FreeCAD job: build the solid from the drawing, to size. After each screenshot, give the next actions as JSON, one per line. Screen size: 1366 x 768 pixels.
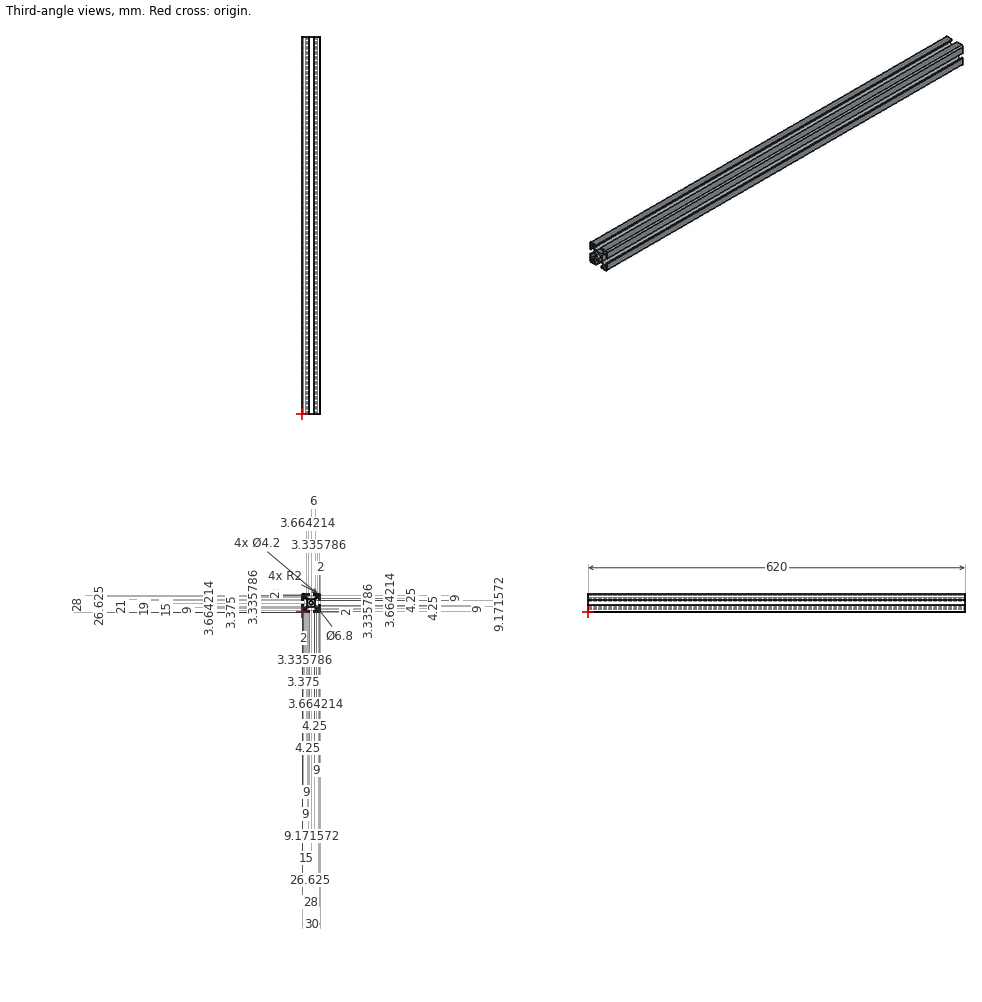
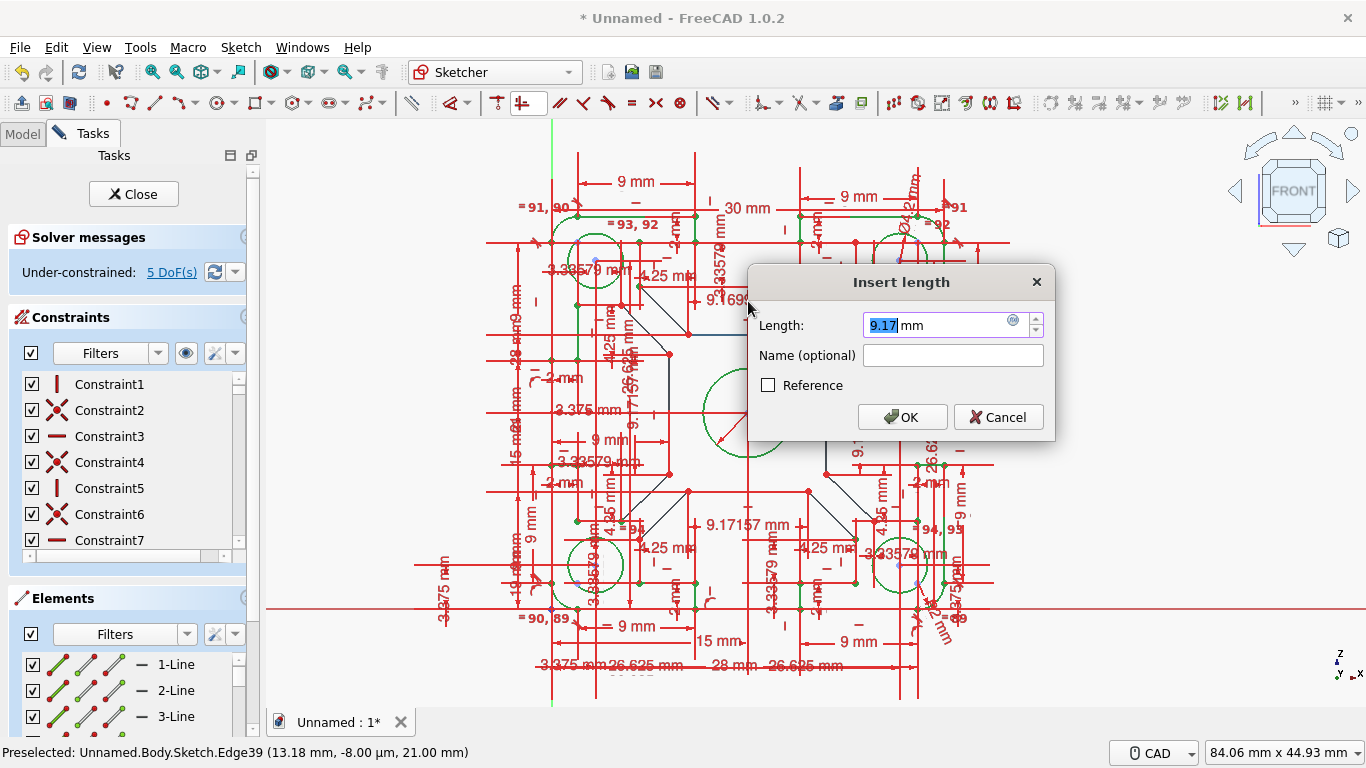
{"action": "type", "text": "9.171572"}
{"action": "key", "text": "Return"}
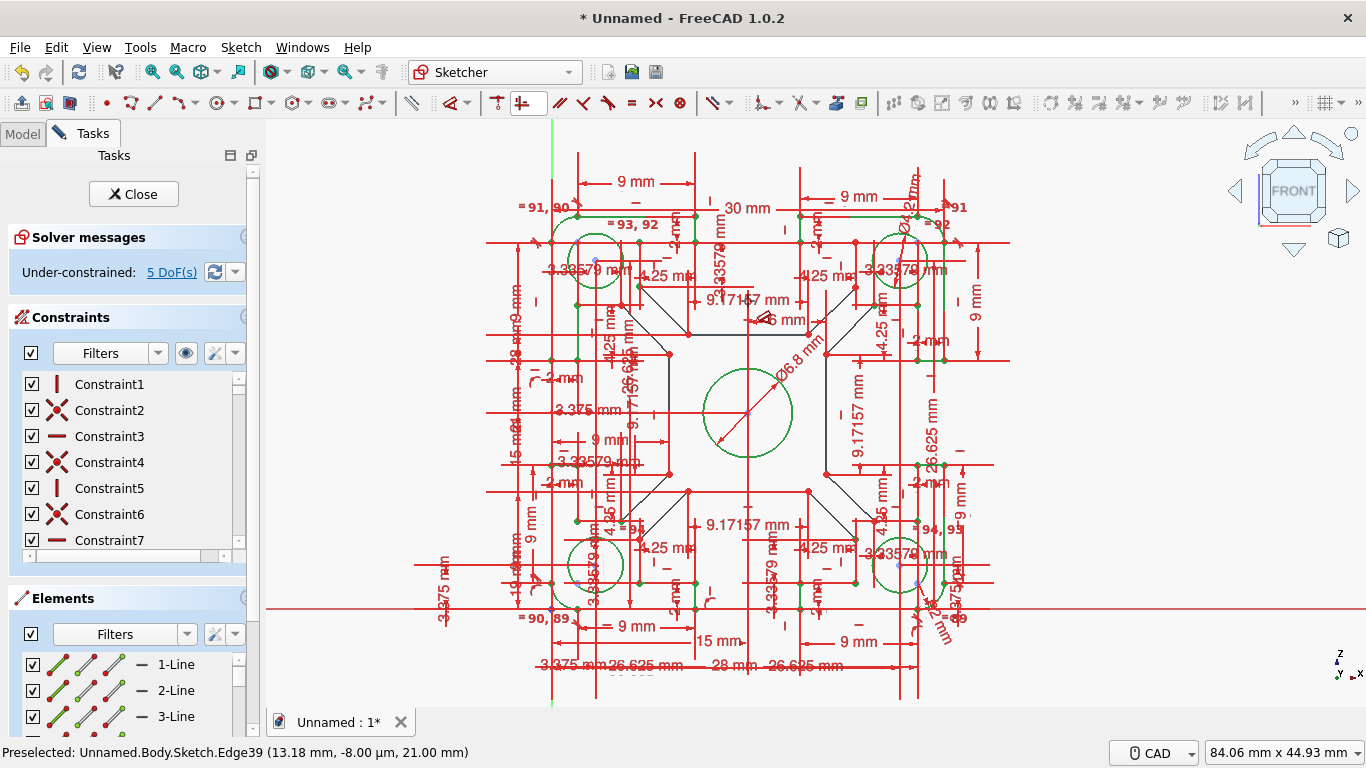
{"action": "left_click", "coordinate": [856, 274]}
{"action": "left_click", "coordinate": [962, 250]}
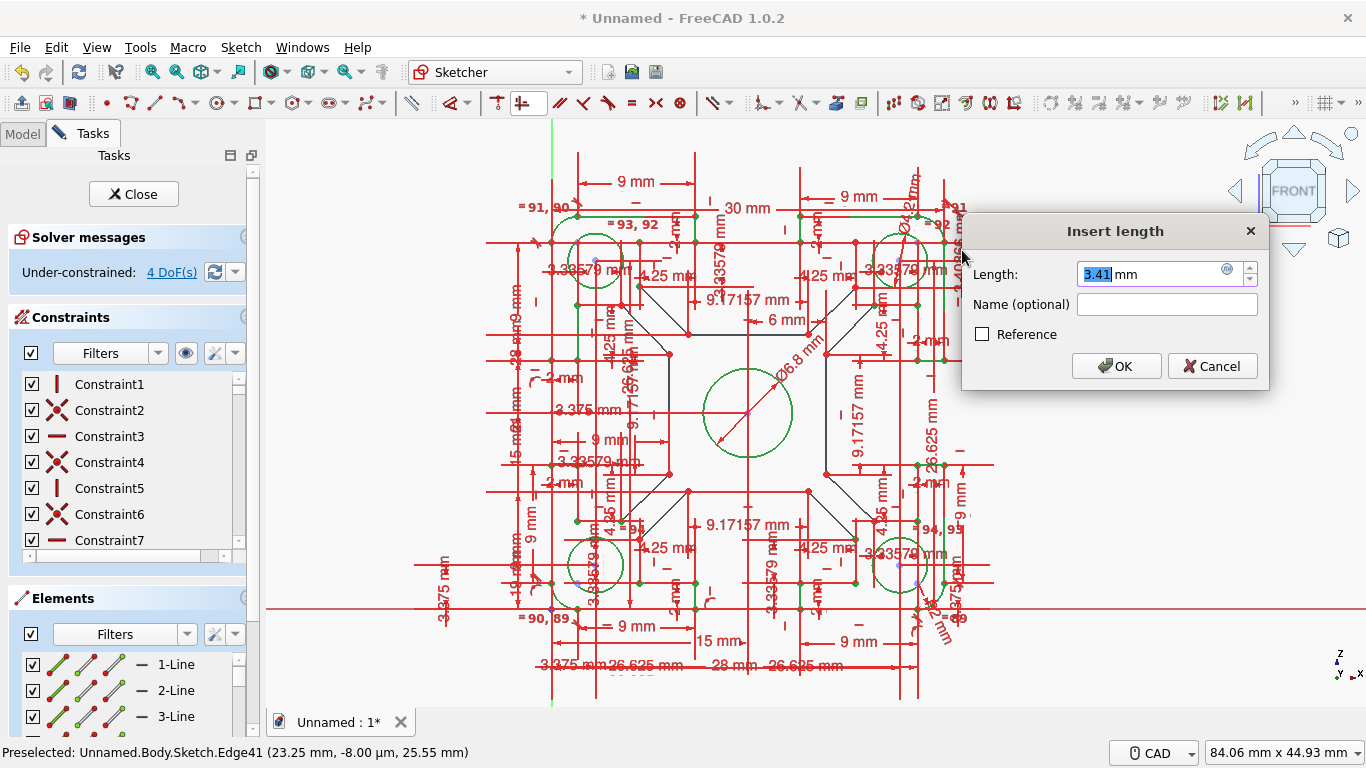
{"action": "type", "text": "3.335786"}
{"action": "key", "text": "Return"}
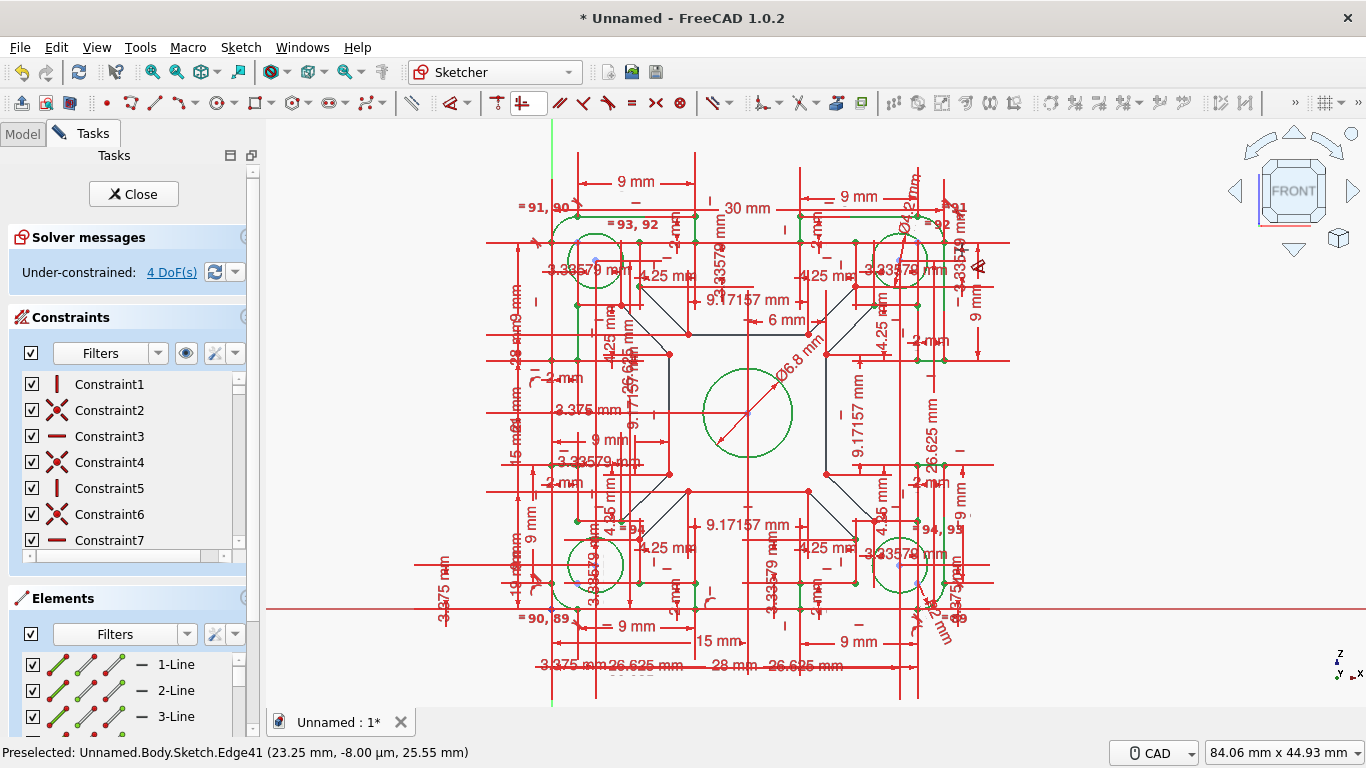
{"action": "left_click", "coordinate": [860, 320]}
{"action": "left_click", "coordinate": [1004, 330]}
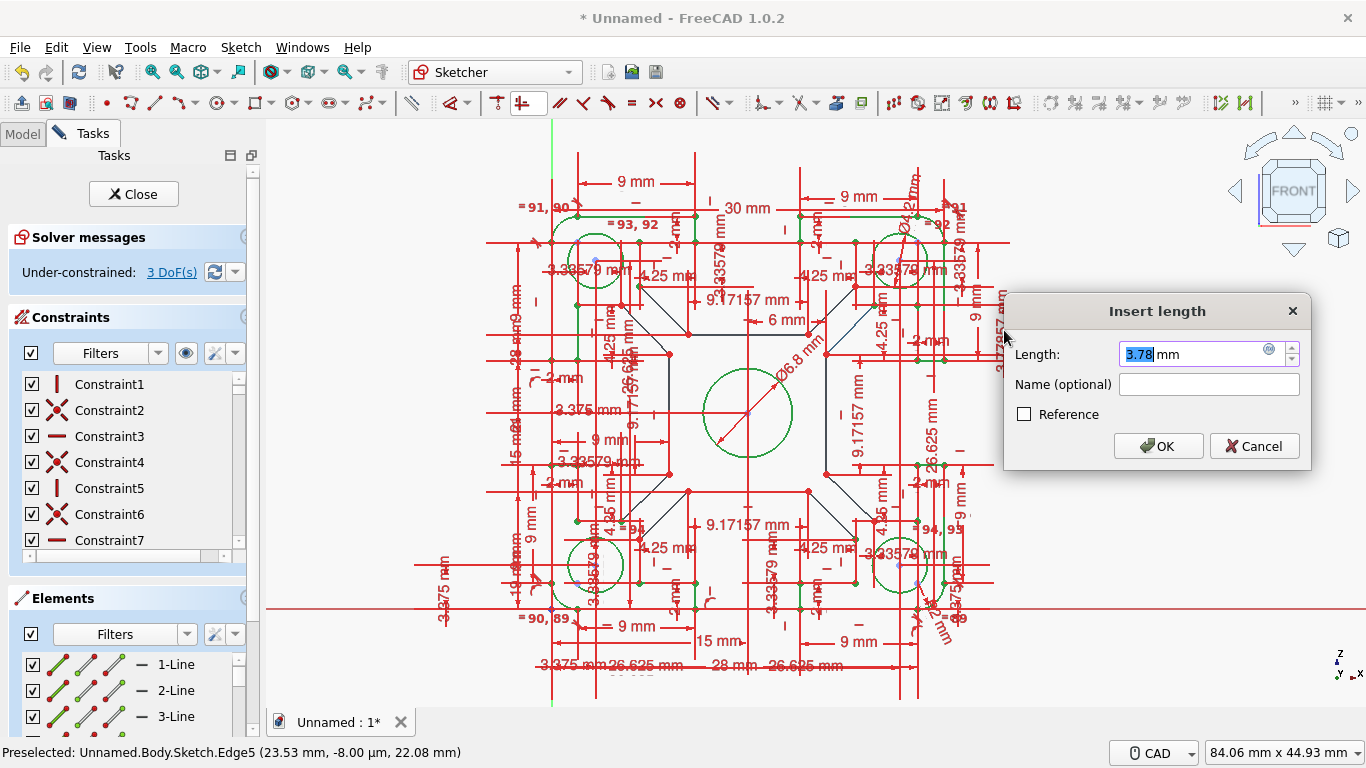
{"action": "type", "text": "3.664214"}
{"action": "key", "text": "Return"}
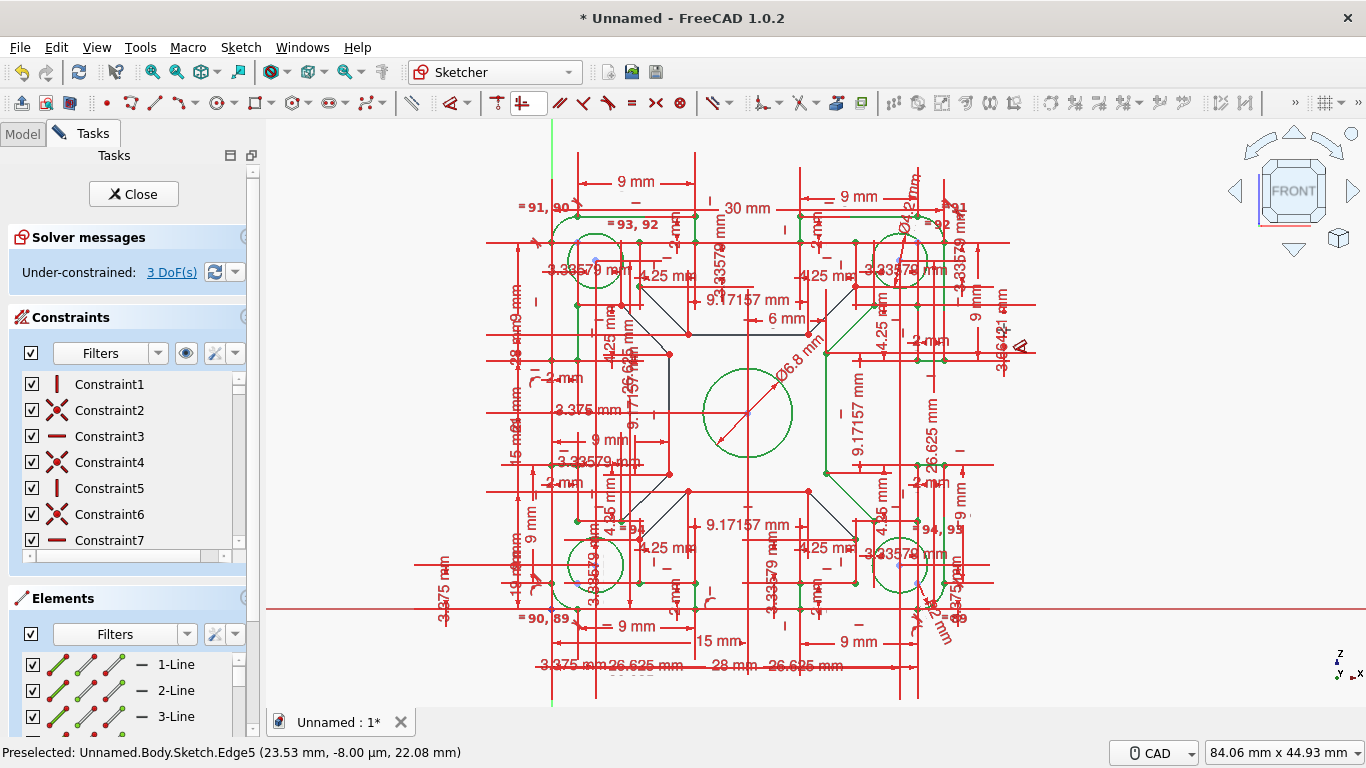
{"action": "left_click", "coordinate": [841, 525]}
{"action": "left_click", "coordinate": [843, 458]}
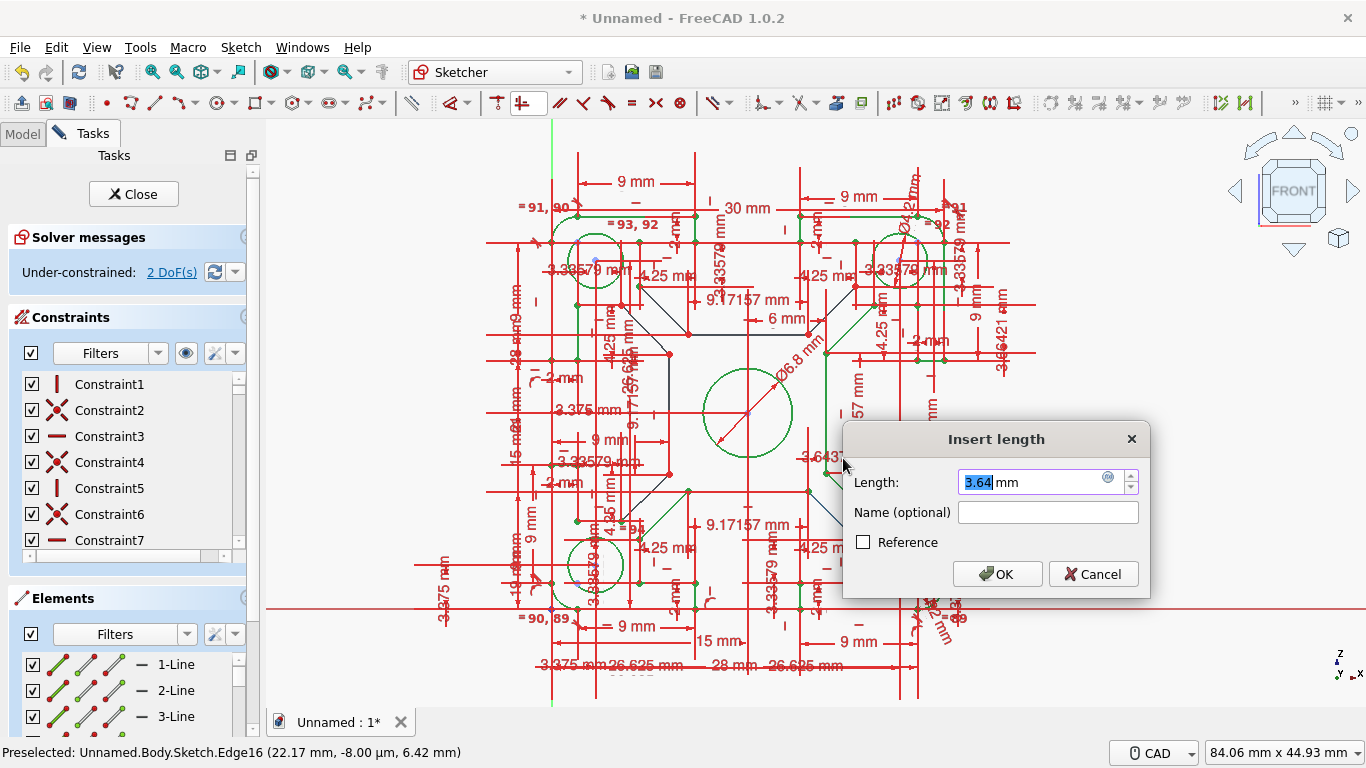
{"action": "type", "text": "3.664214"}
{"action": "key", "text": "Return"}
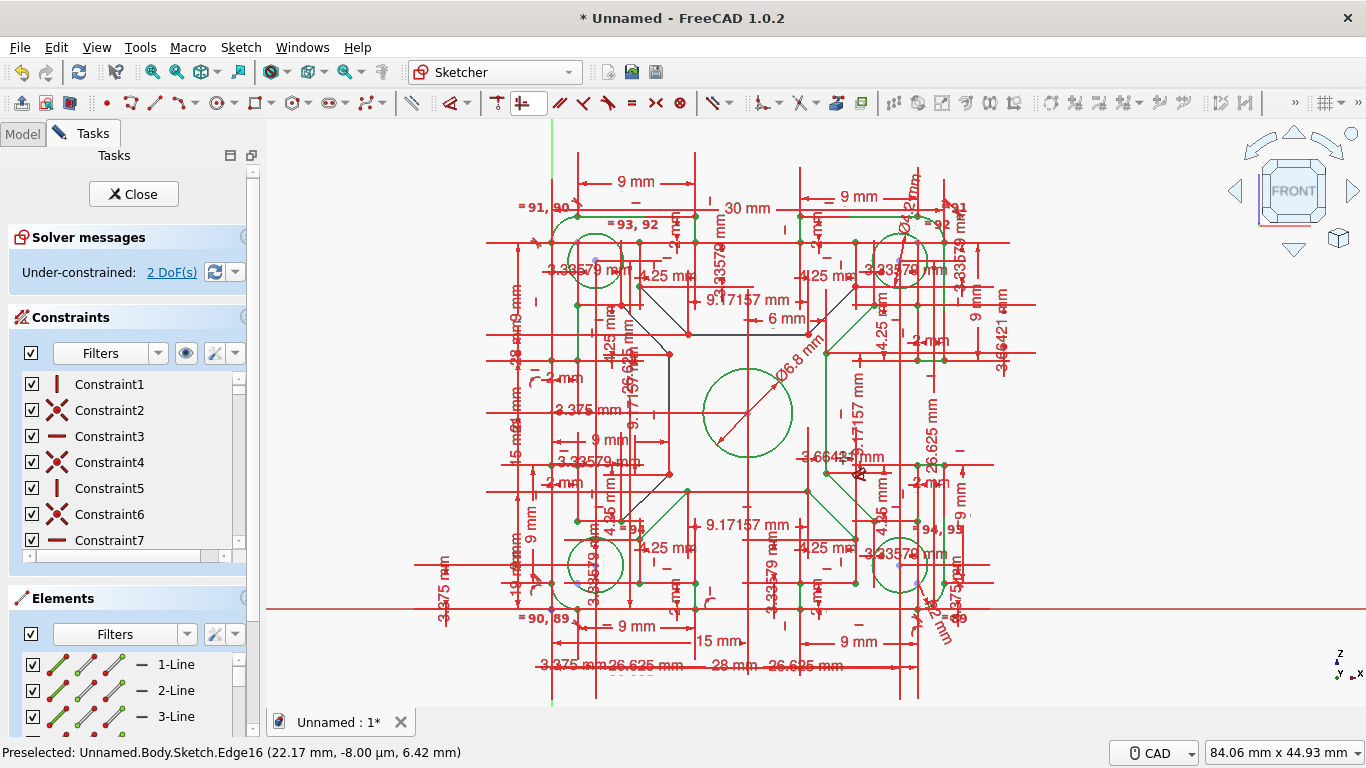
{"action": "left_click", "coordinate": [636, 507]}
{"action": "left_click", "coordinate": [491, 498]}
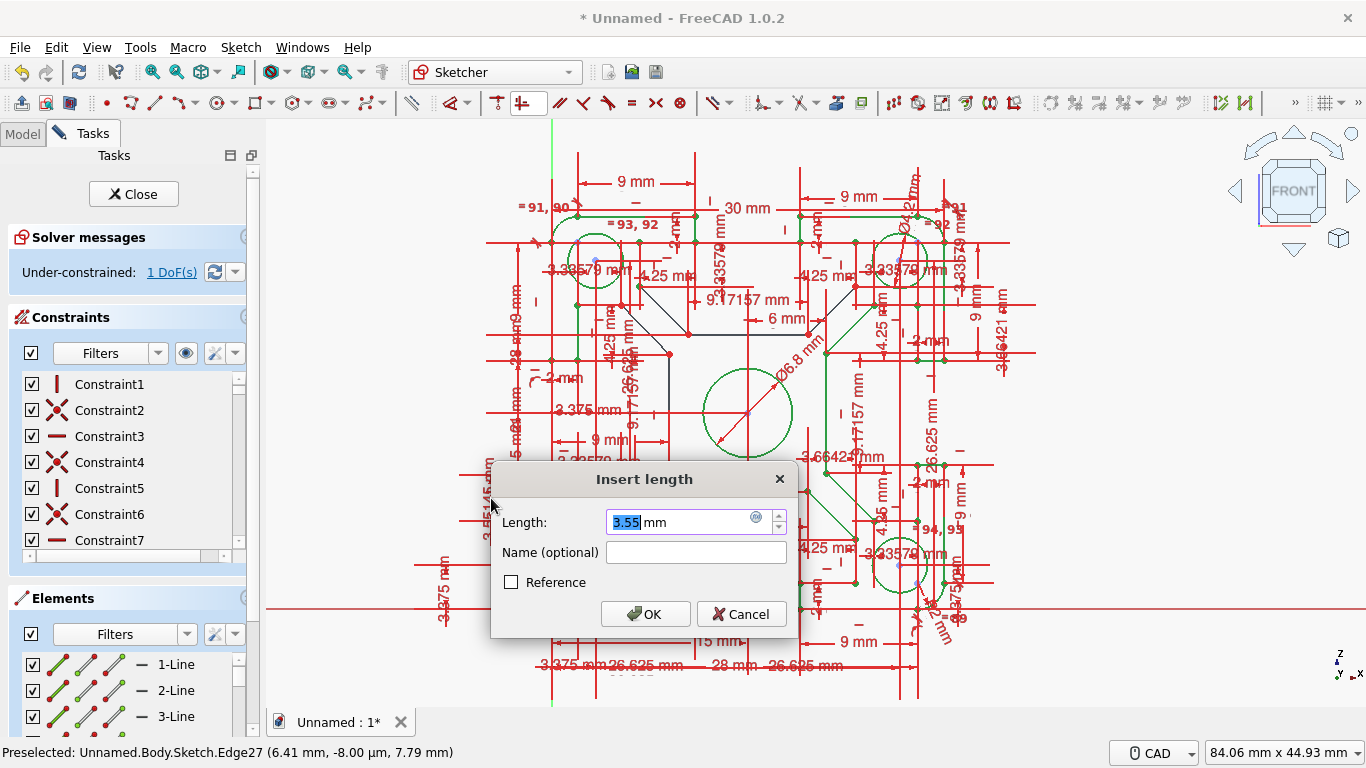
{"action": "type", "text": "3.664214"}
{"action": "key", "text": "Return"}